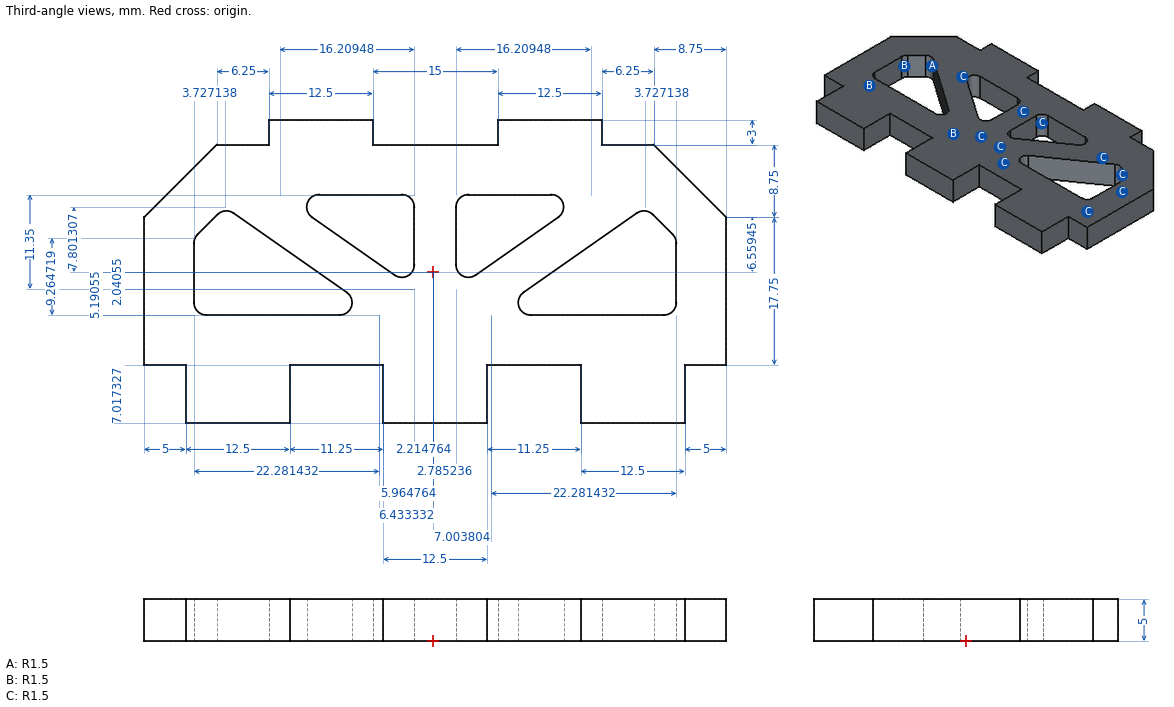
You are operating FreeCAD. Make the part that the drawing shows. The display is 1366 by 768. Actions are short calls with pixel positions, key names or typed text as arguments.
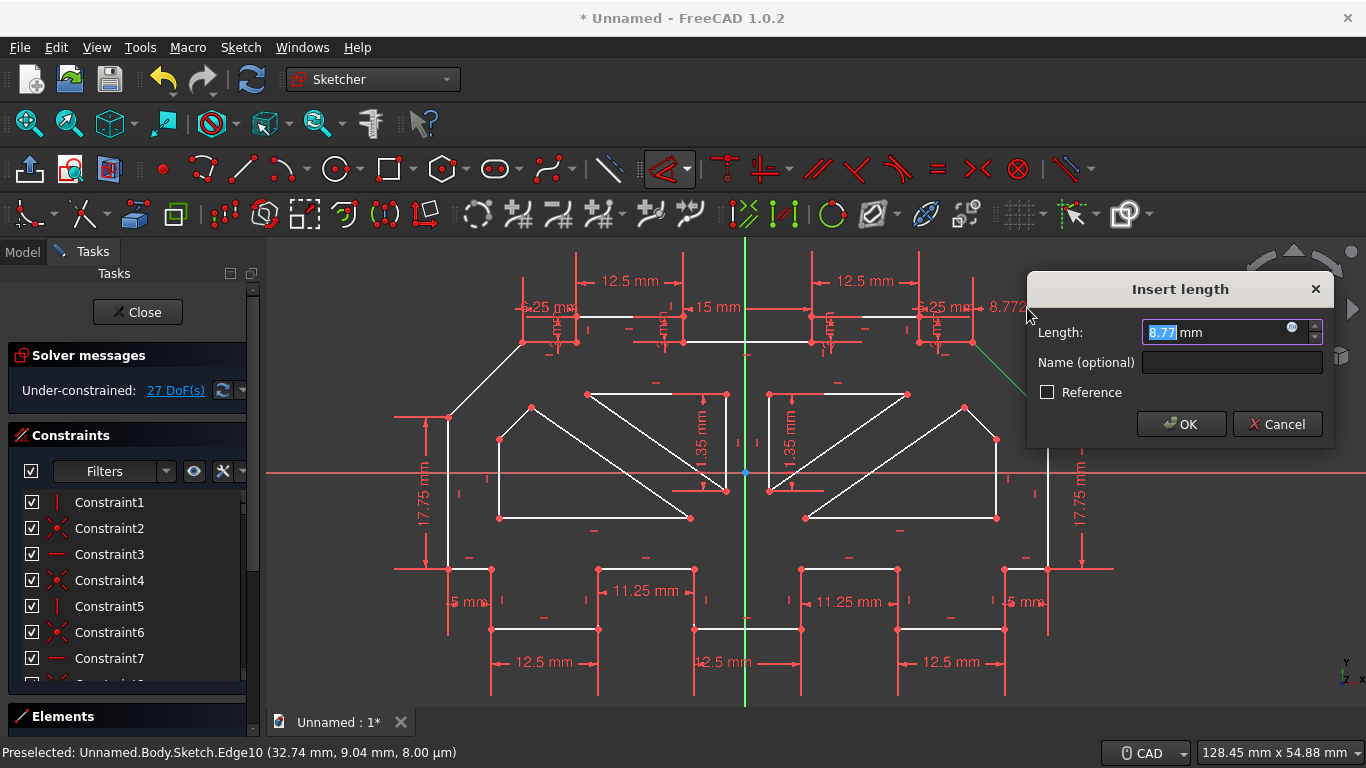
text(8.75)
key(Return)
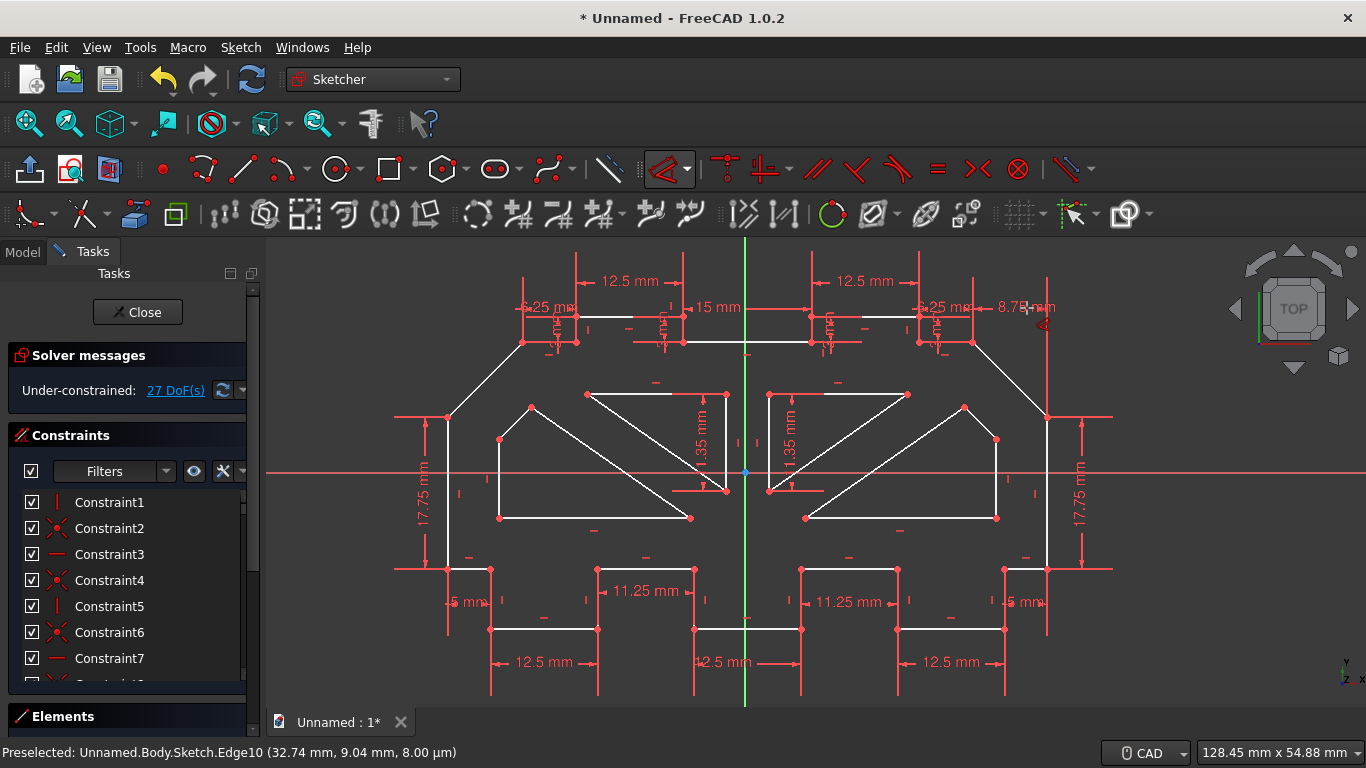
click(1025, 395)
click(1081, 380)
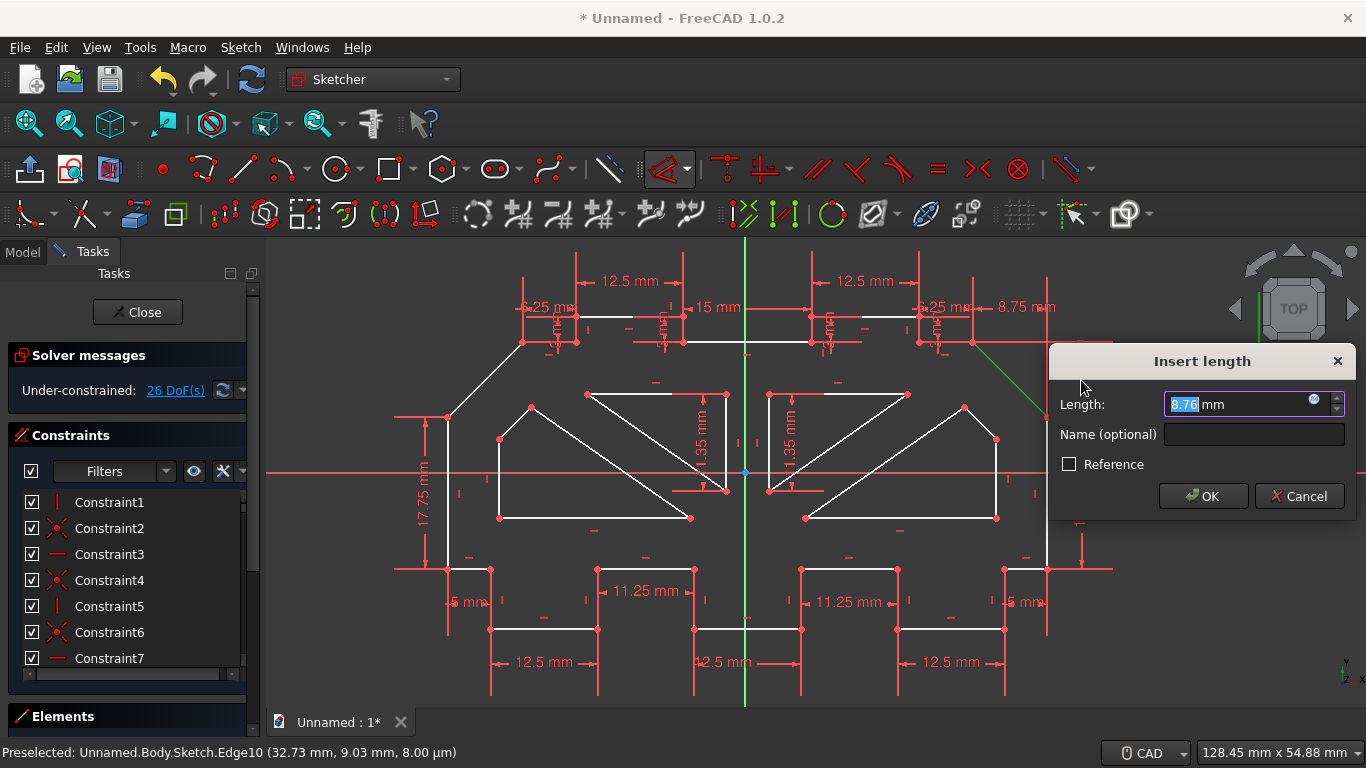
text(8.75)
key(Return)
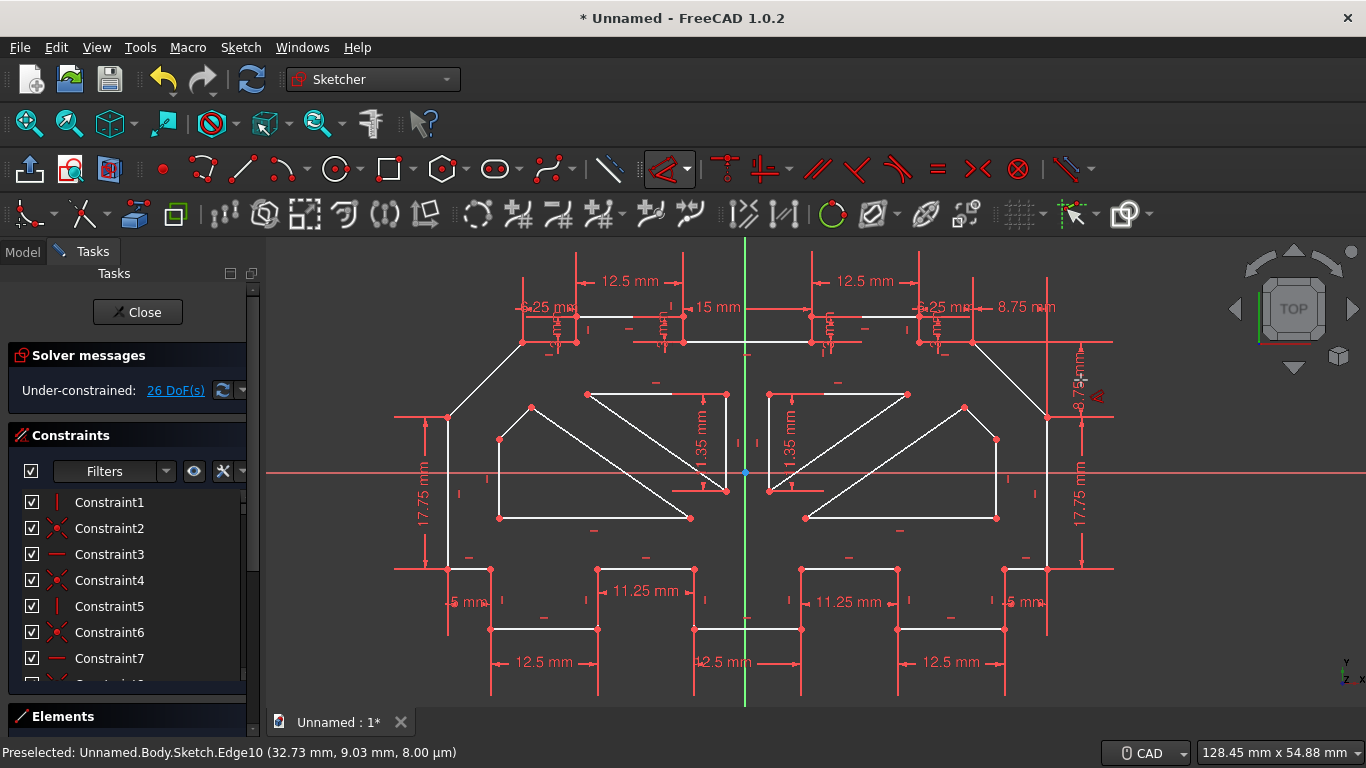
click(500, 365)
click(414, 380)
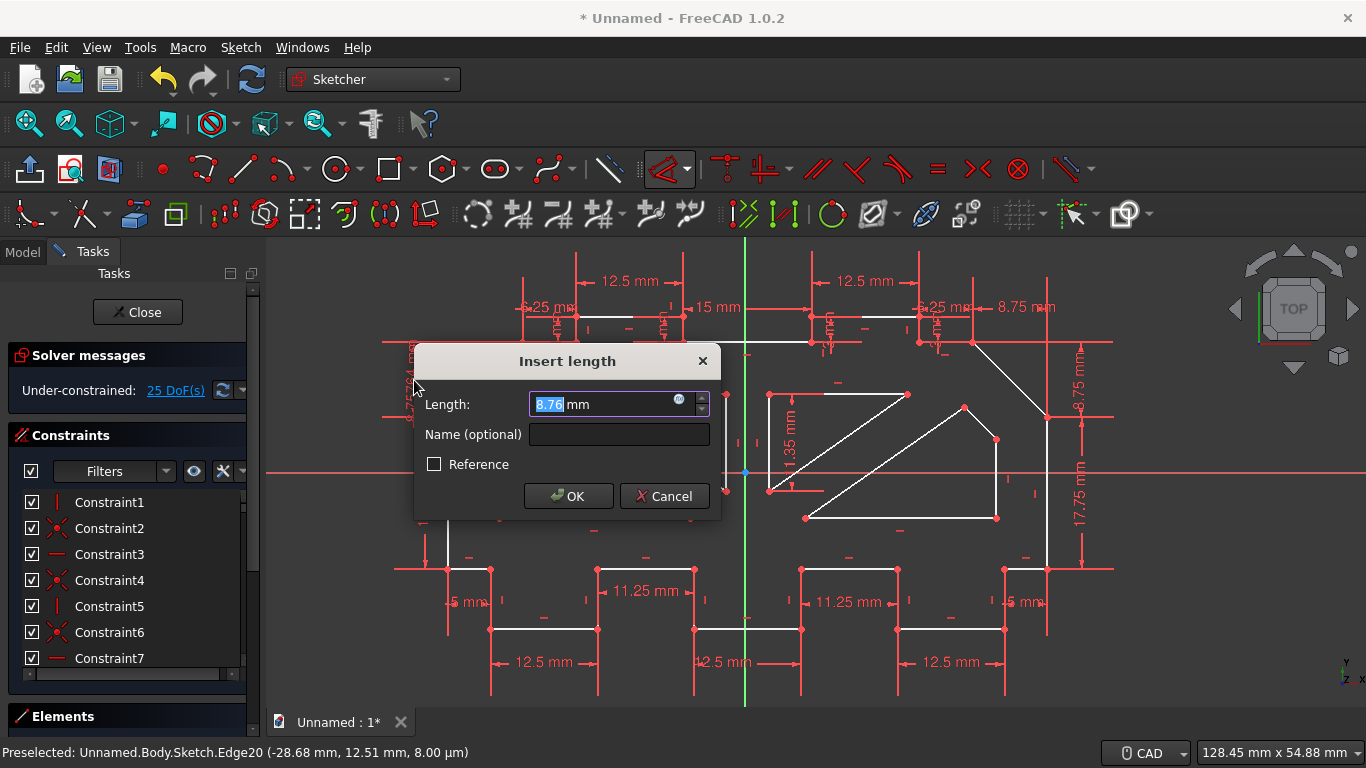
text(8.75)
key(Return)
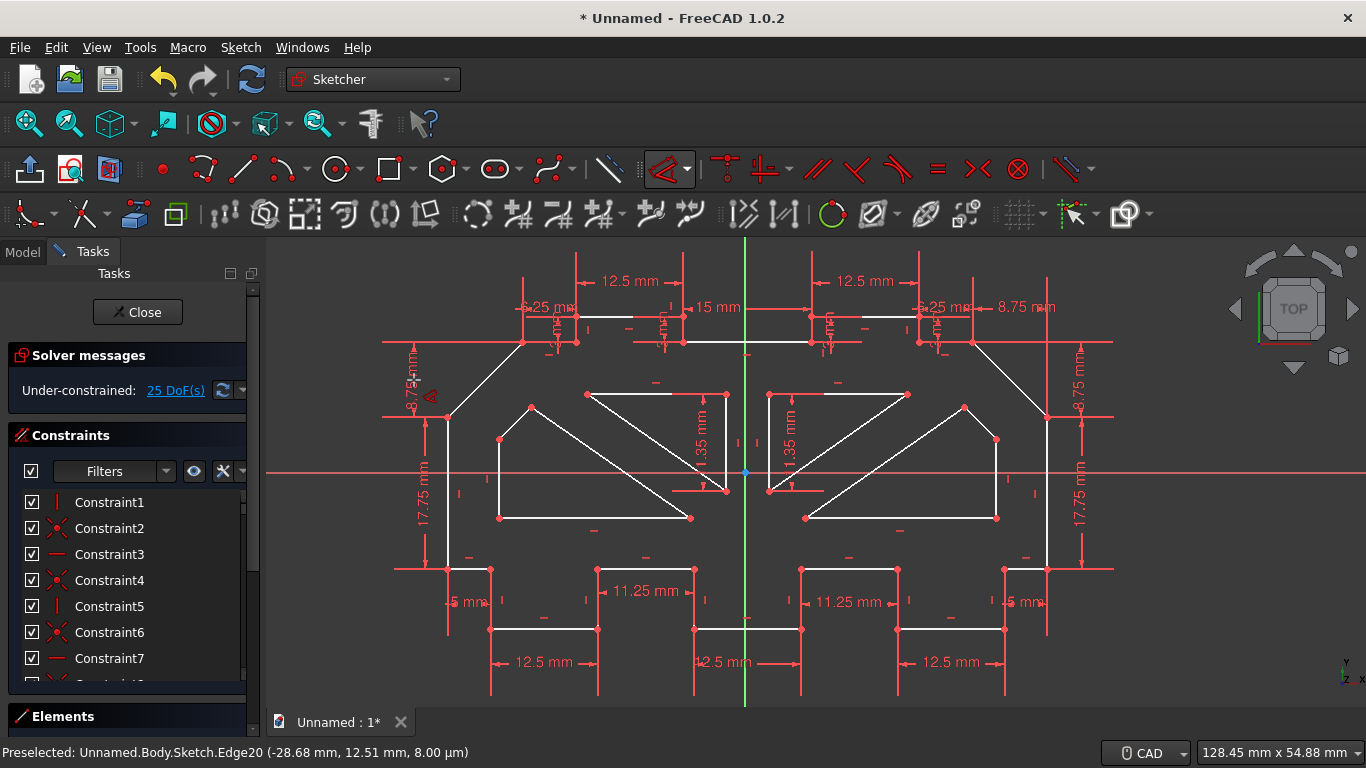
click(694, 587)
click(660, 613)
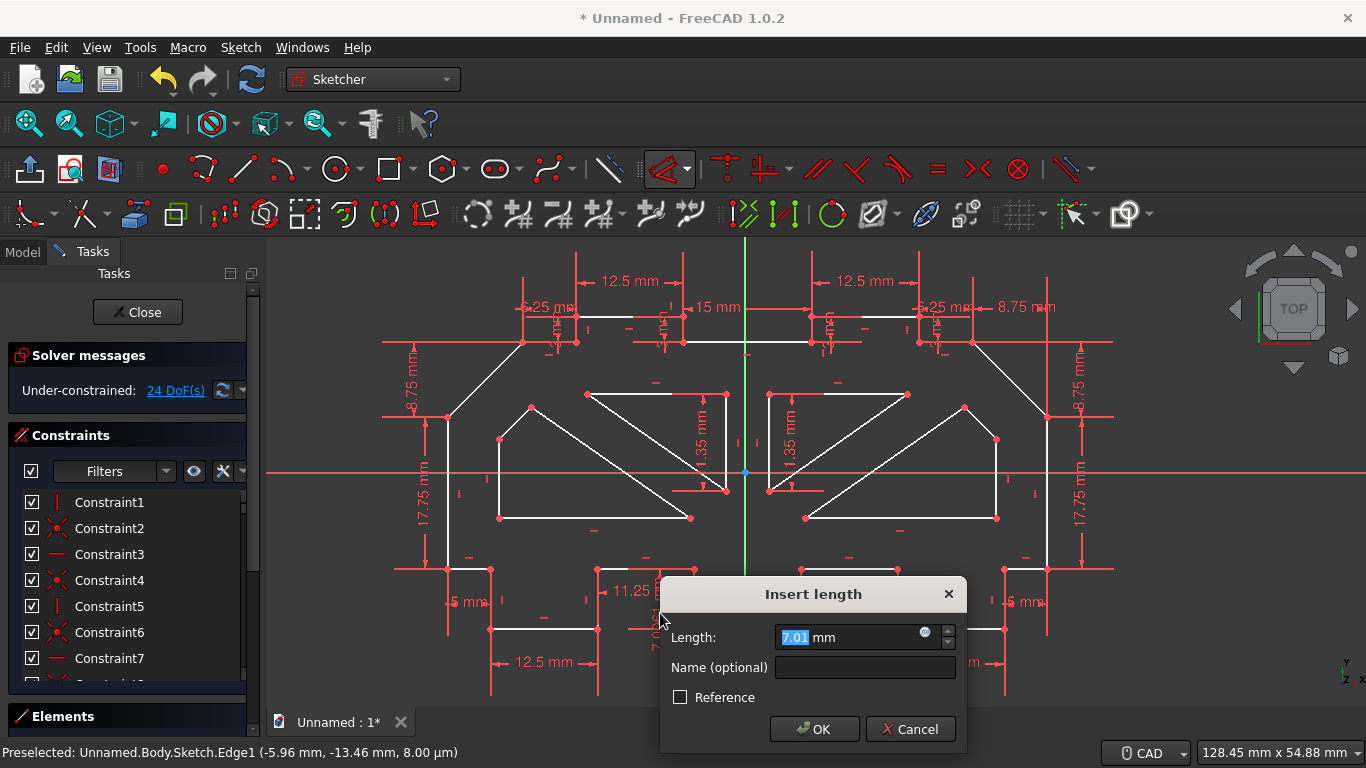
text(7.017327)
key(Return)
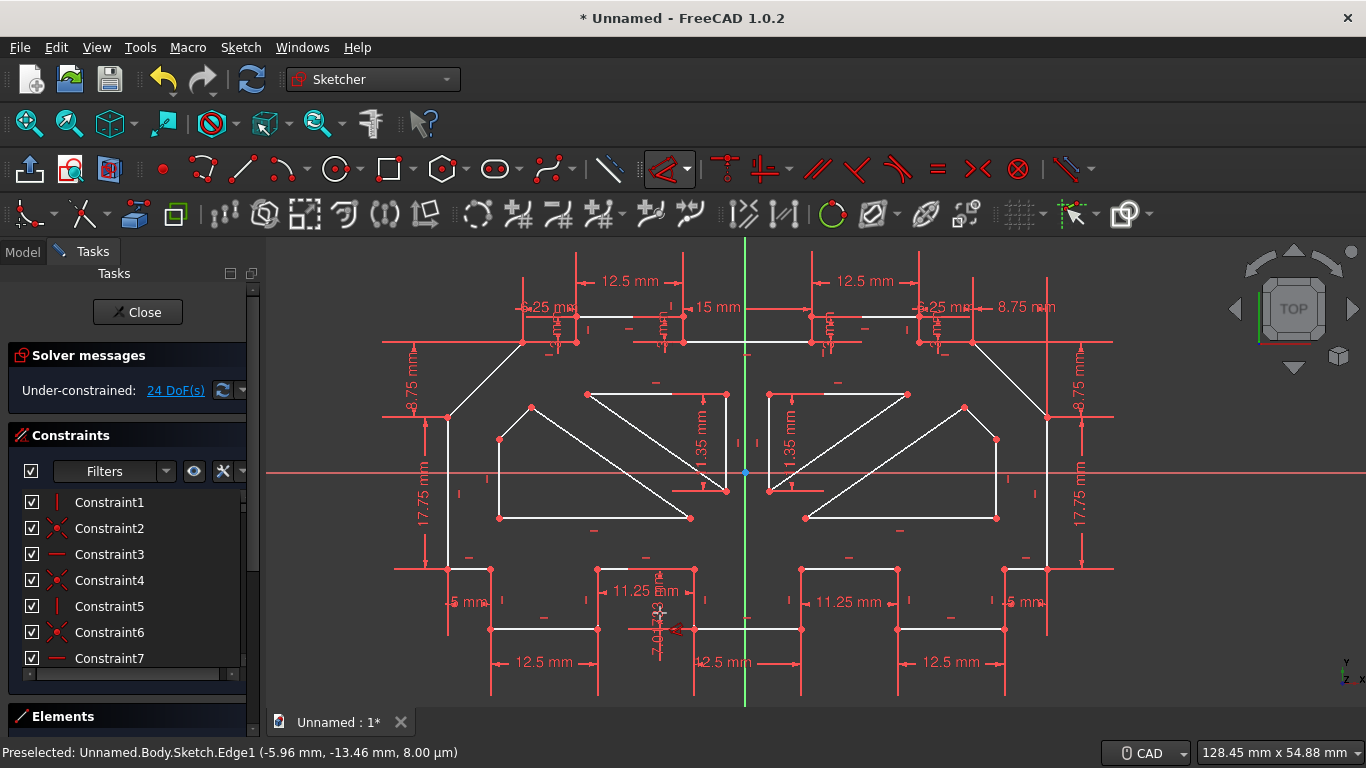
click(801, 611)
click(767, 599)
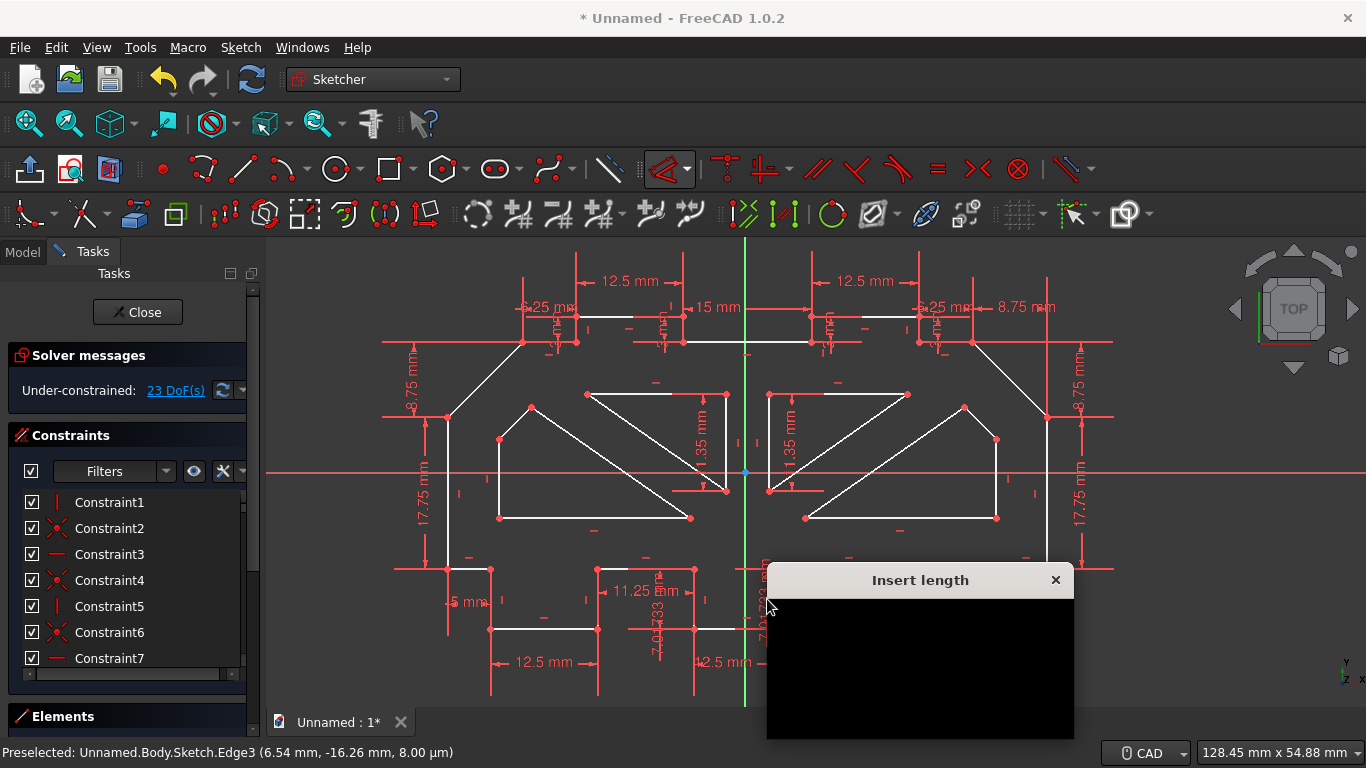
text(7.017327)
key(Return)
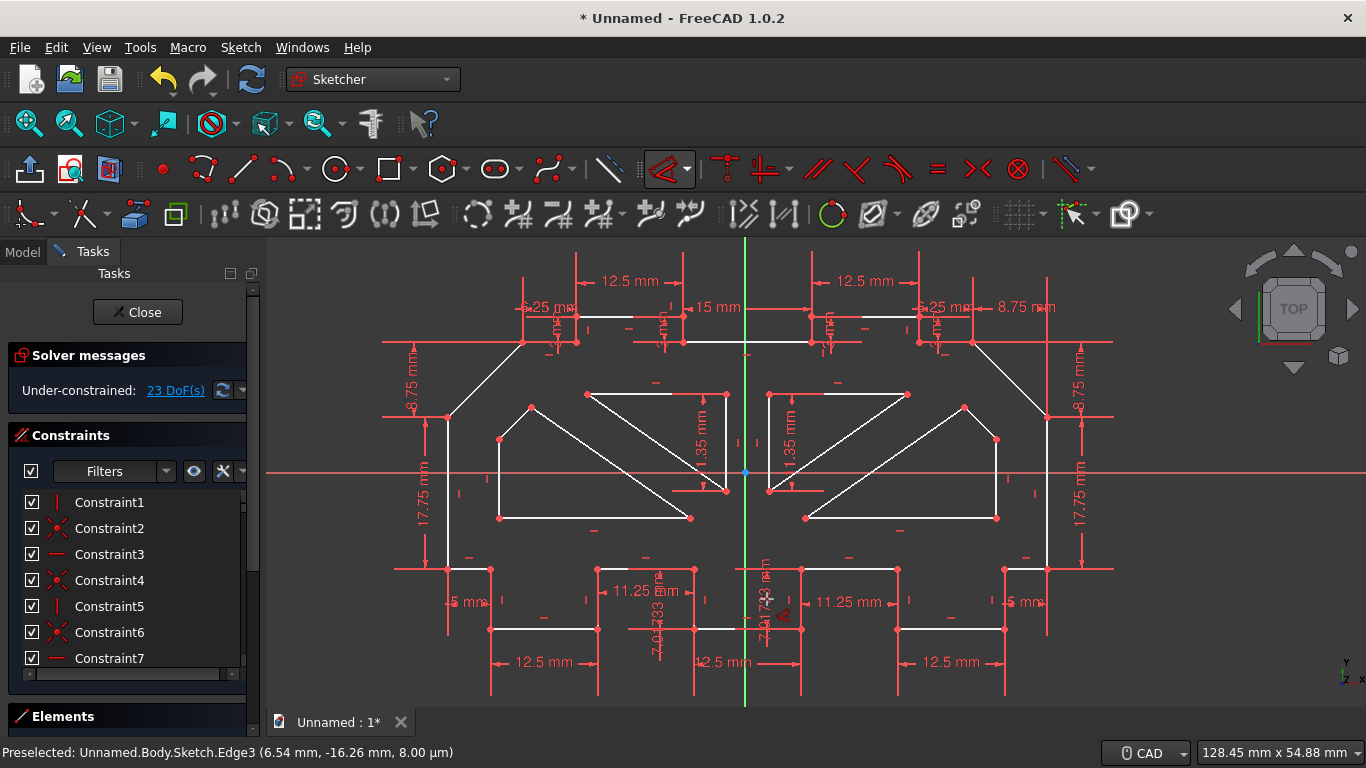
click(898, 587)
click(932, 599)